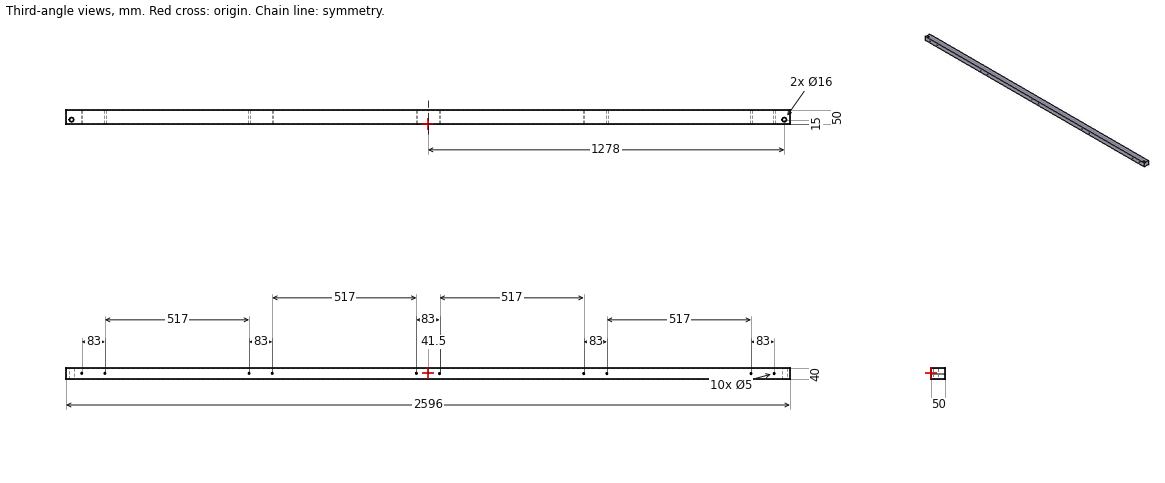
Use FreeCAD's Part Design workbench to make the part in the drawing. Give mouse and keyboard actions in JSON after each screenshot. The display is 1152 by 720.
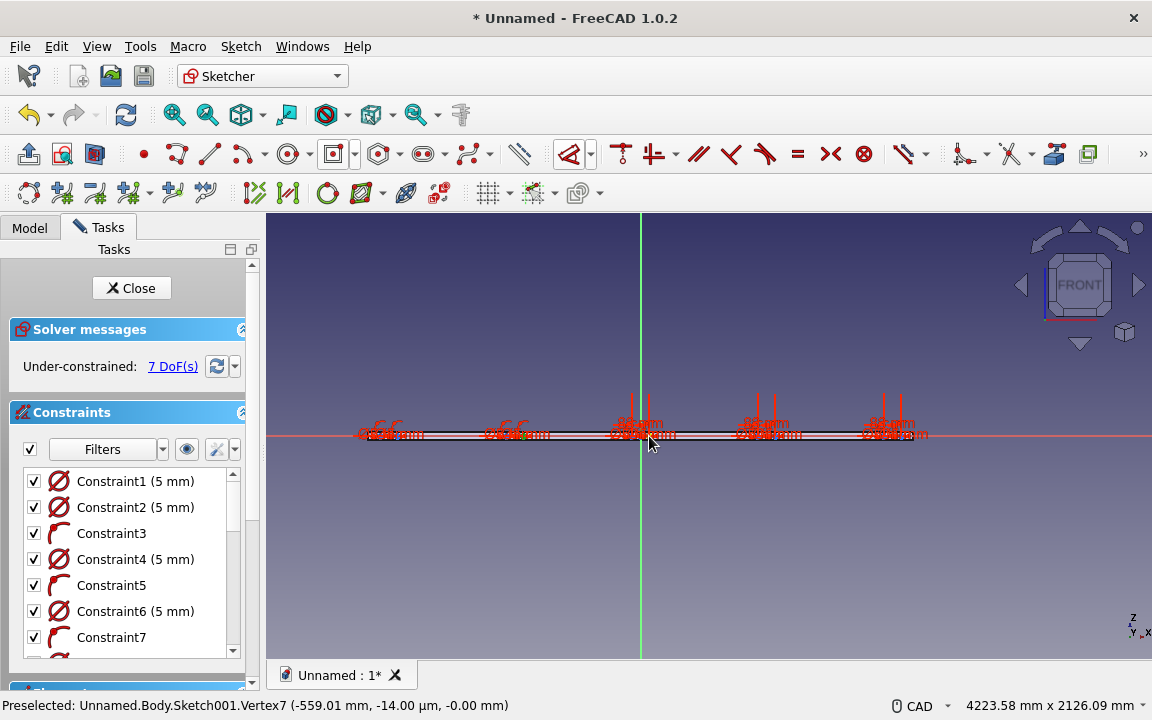
{"action": "scroll", "coordinate": [506, 436], "scroll_direction": "up", "scroll_amount": 5}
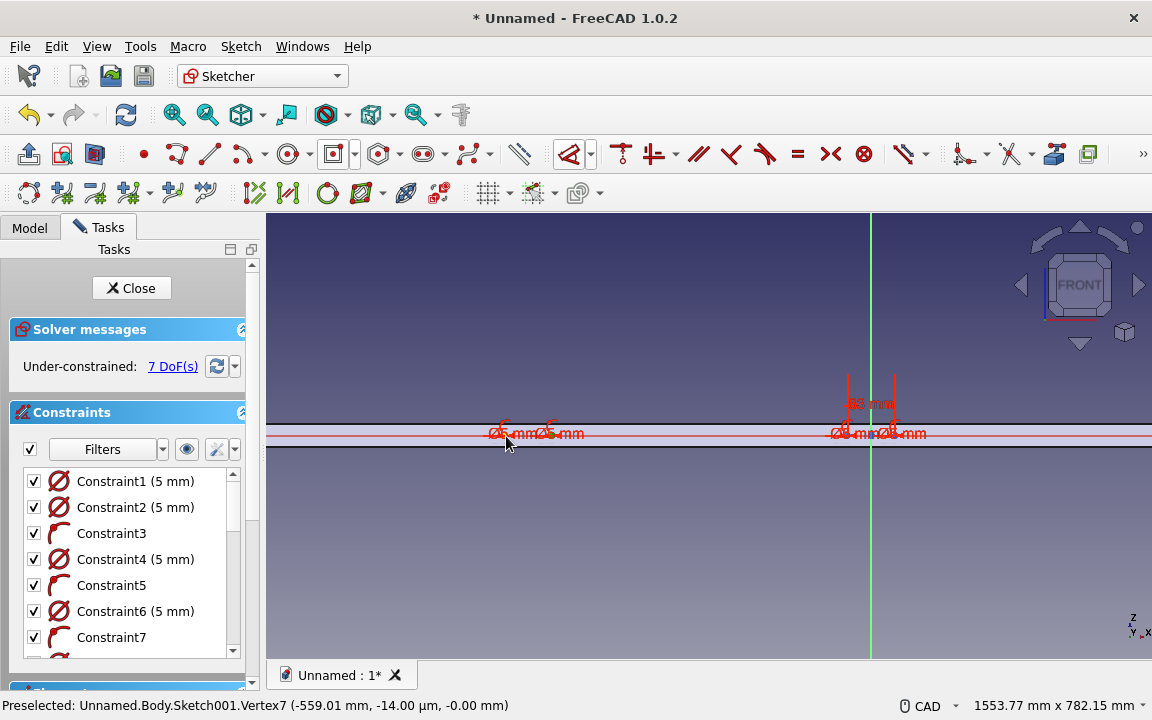
{"action": "left_click", "coordinate": [506, 436]}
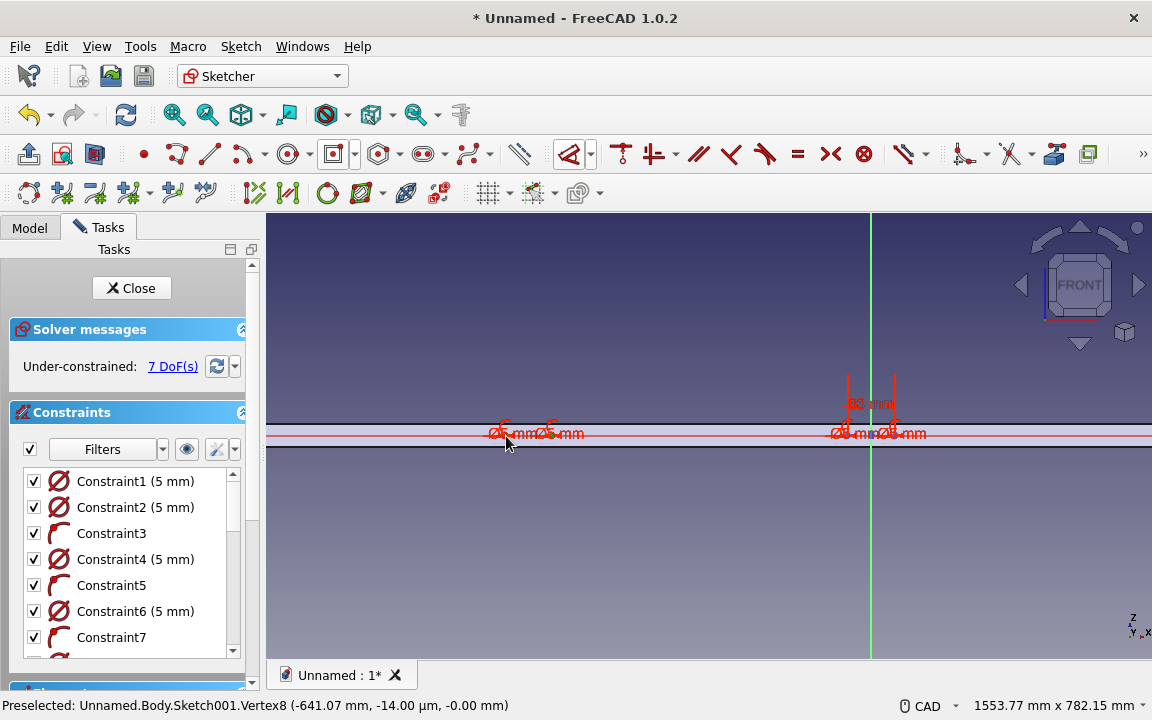
{"action": "left_click", "coordinate": [590, 154]}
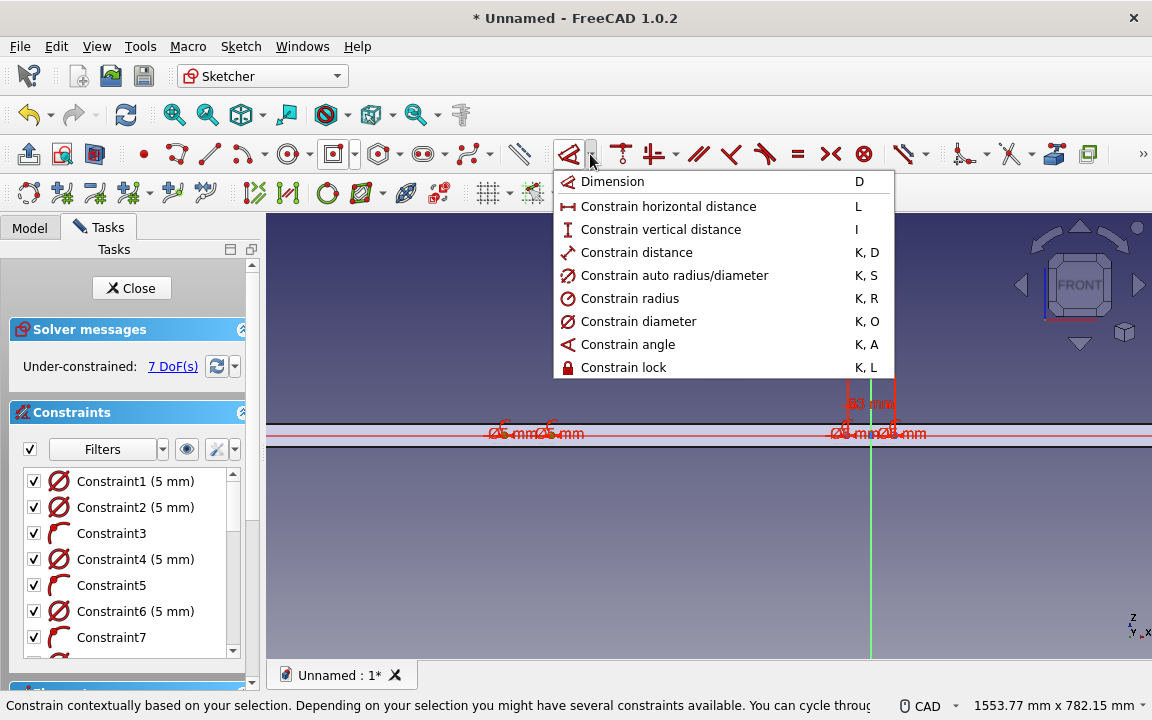
{"action": "left_click", "coordinate": [724, 206]}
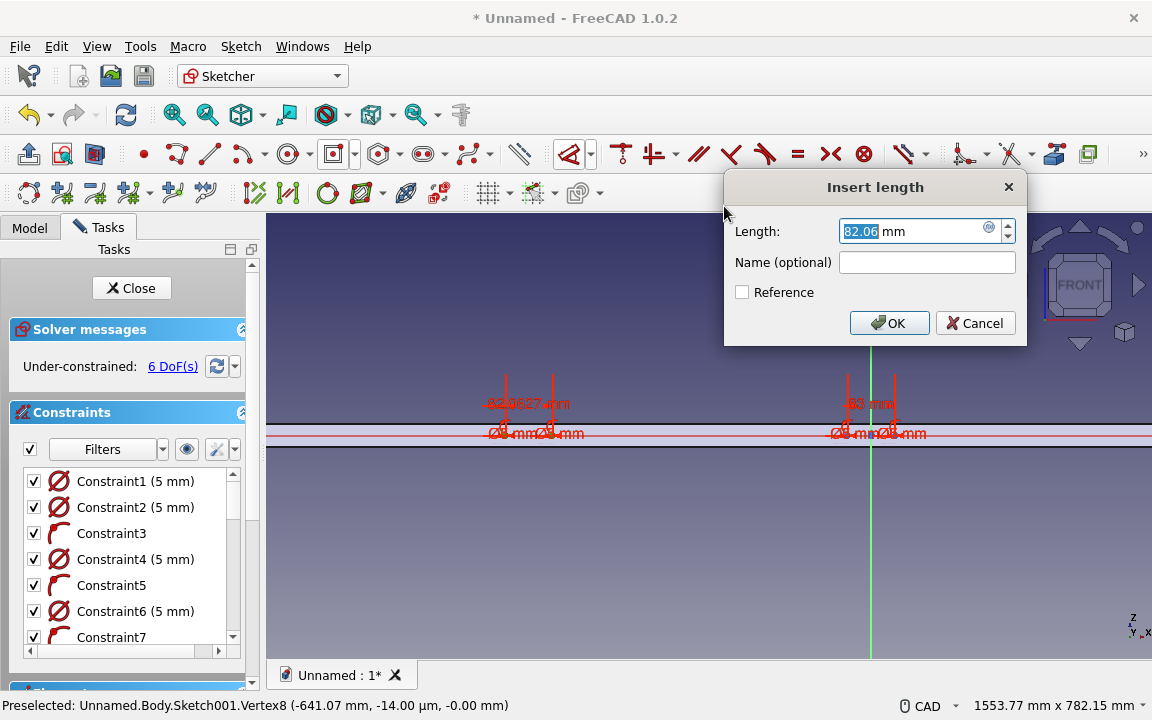
{"action": "type", "text": "83"}
{"action": "key", "text": "Return"}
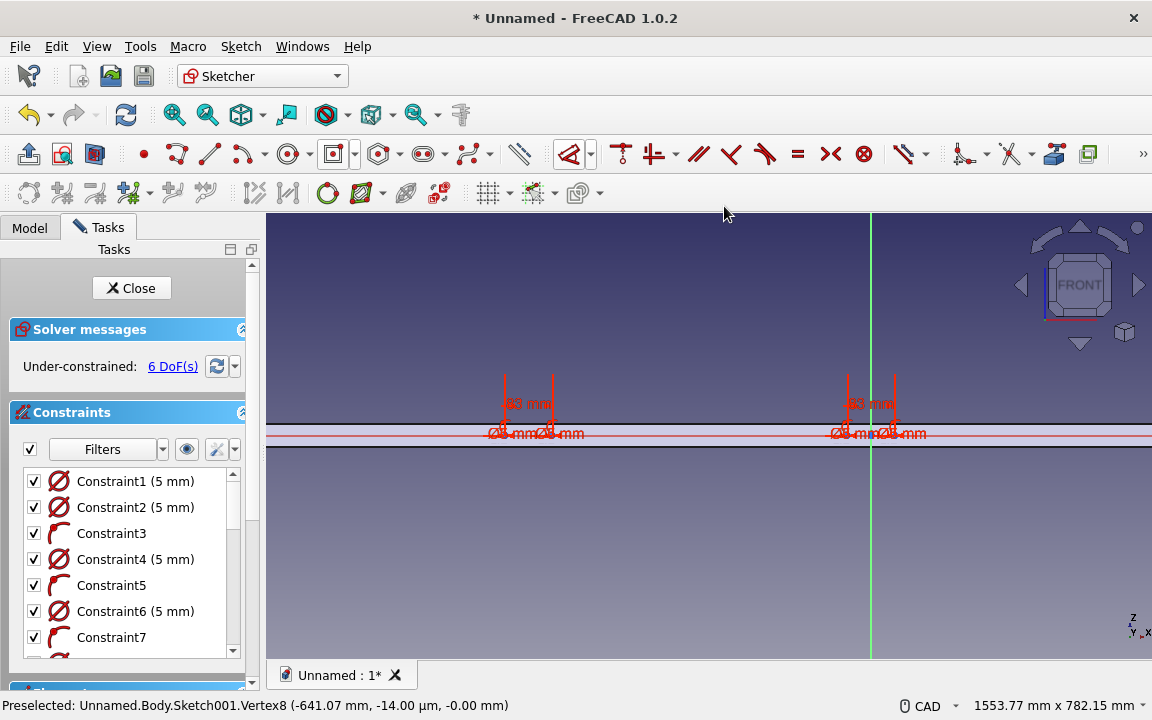
{"action": "scroll", "coordinate": [506, 436], "scroll_direction": "down", "scroll_amount": 5}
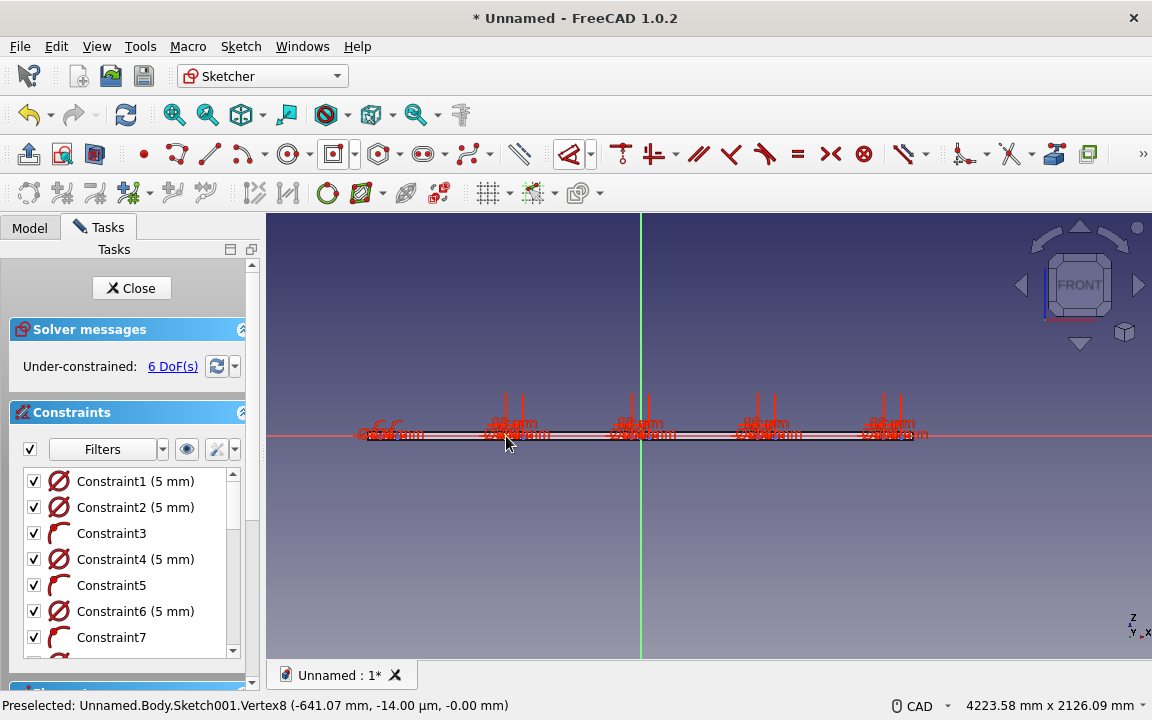
{"action": "scroll", "coordinate": [397, 436], "scroll_direction": "up", "scroll_amount": 5}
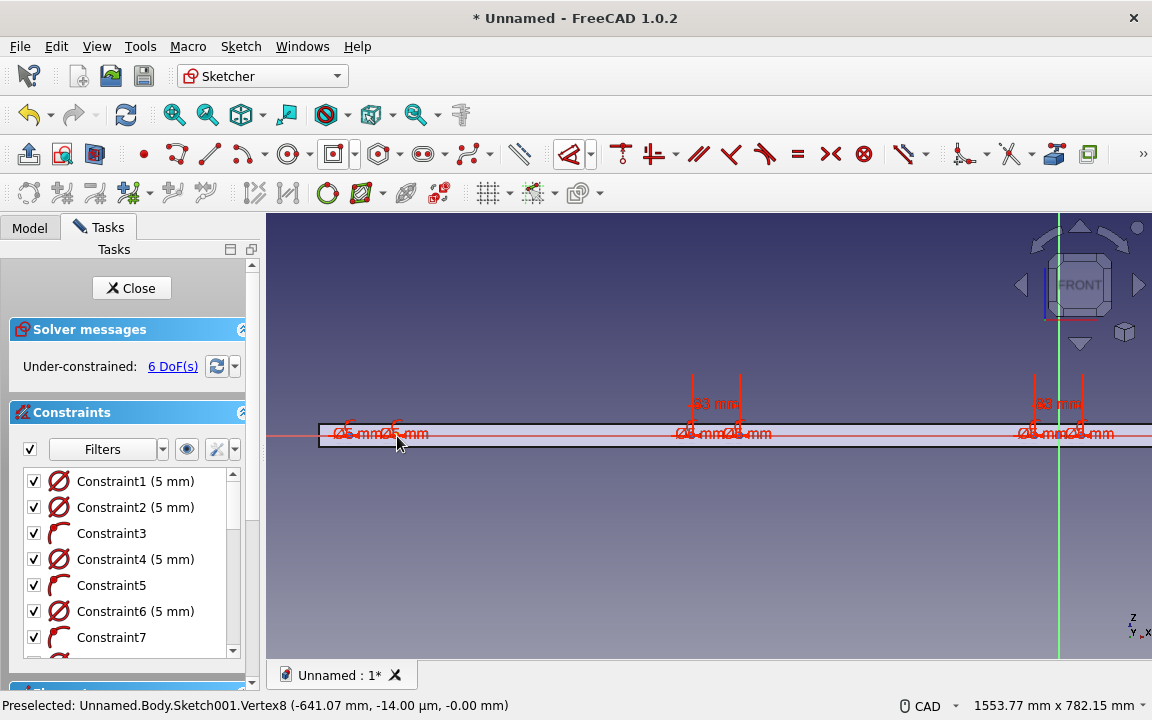
{"action": "left_click", "coordinate": [397, 436]}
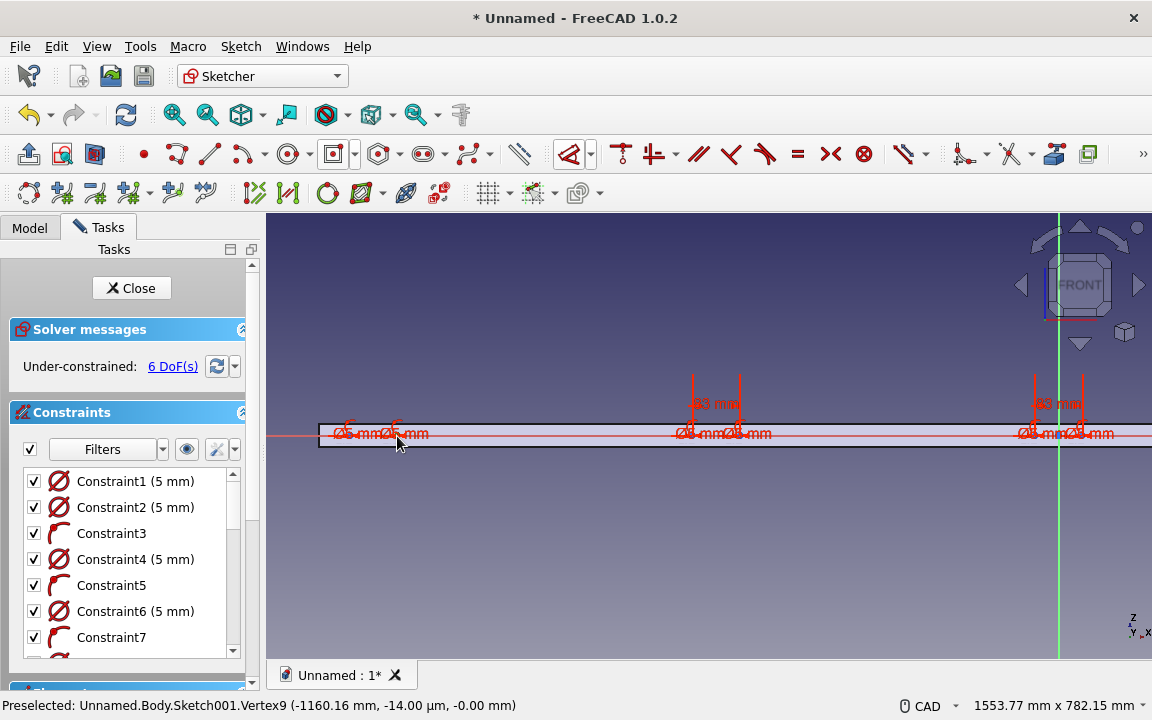
{"action": "left_click", "coordinate": [351, 436]}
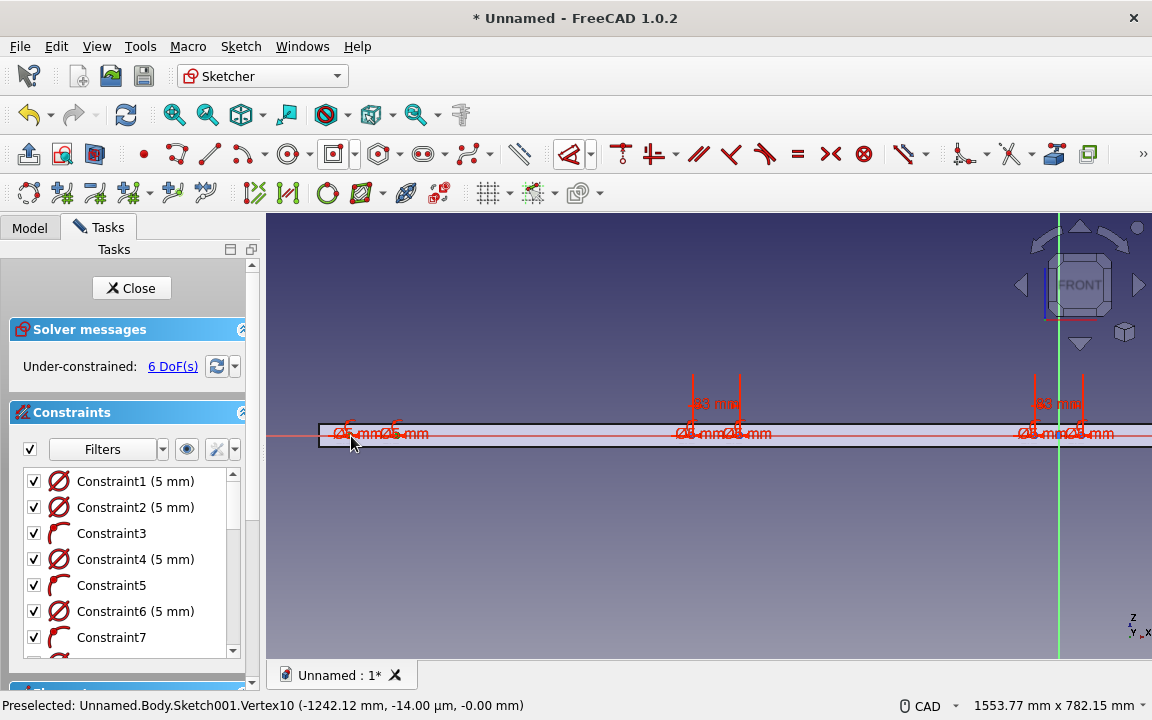
{"action": "key", "text": "l"}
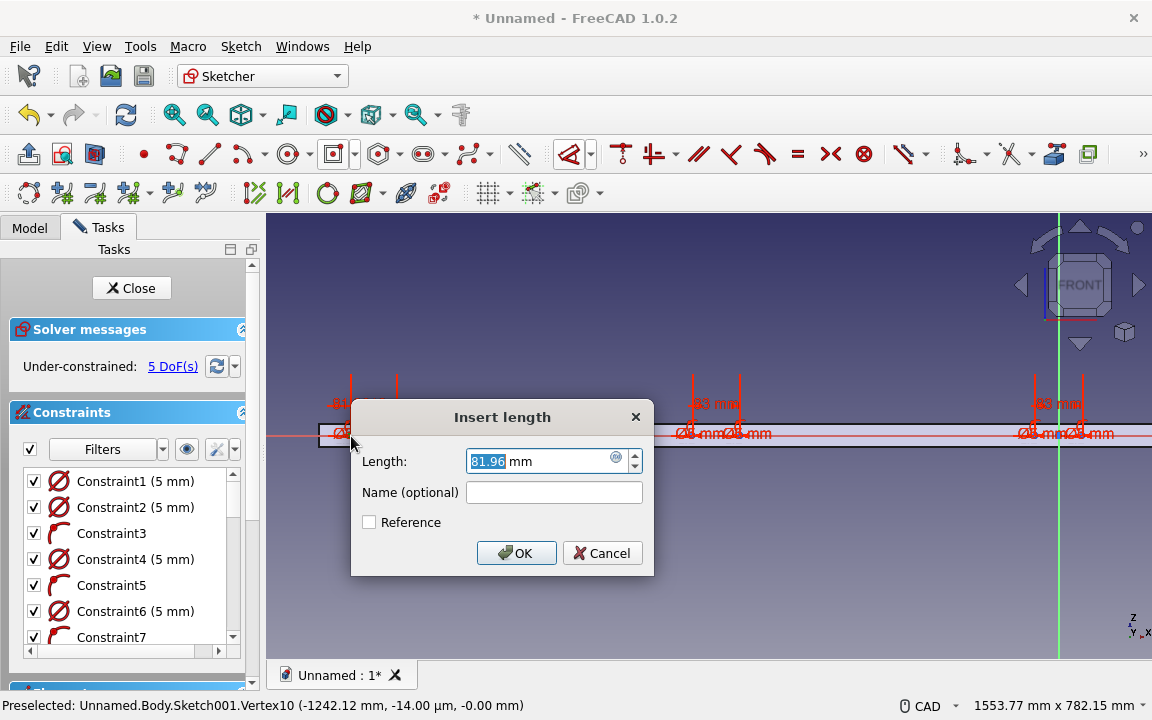
{"action": "type", "text": "83"}
{"action": "key", "text": "Return"}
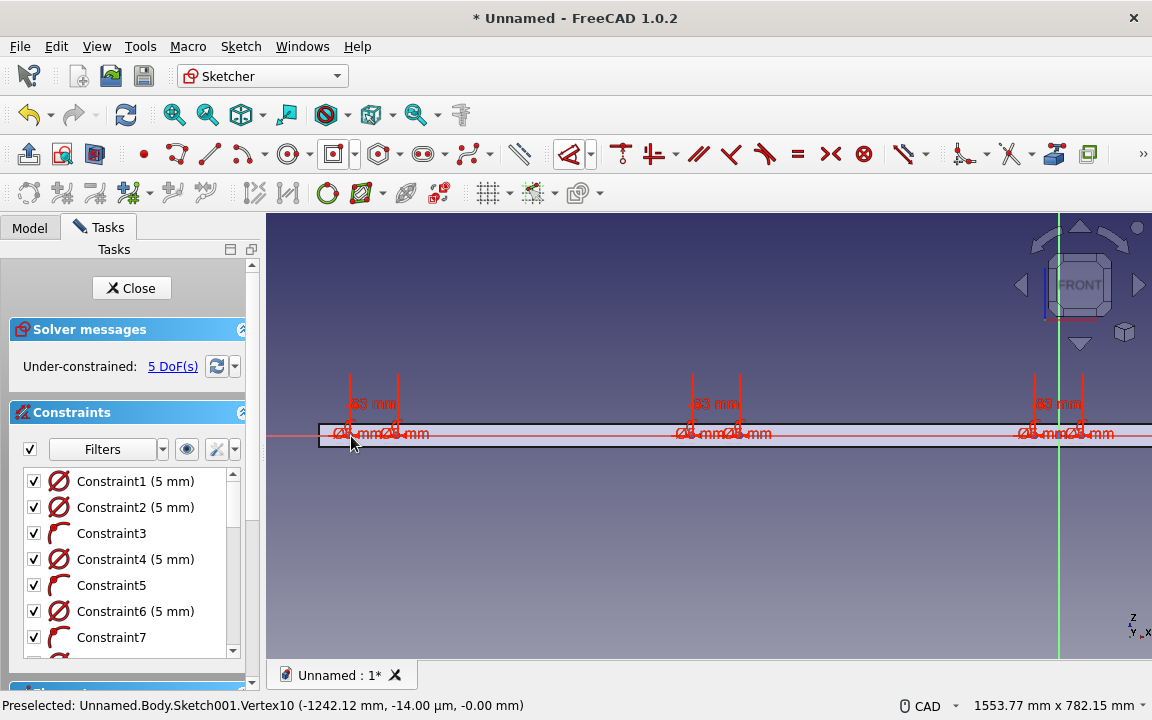
{"action": "scroll", "coordinate": [397, 436], "scroll_direction": "down", "scroll_amount": 5}